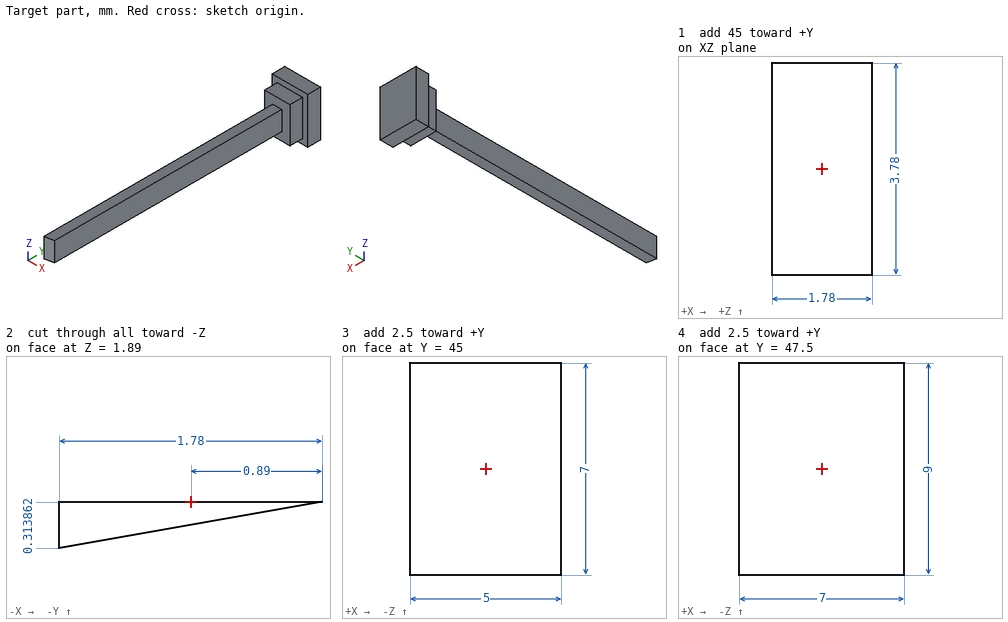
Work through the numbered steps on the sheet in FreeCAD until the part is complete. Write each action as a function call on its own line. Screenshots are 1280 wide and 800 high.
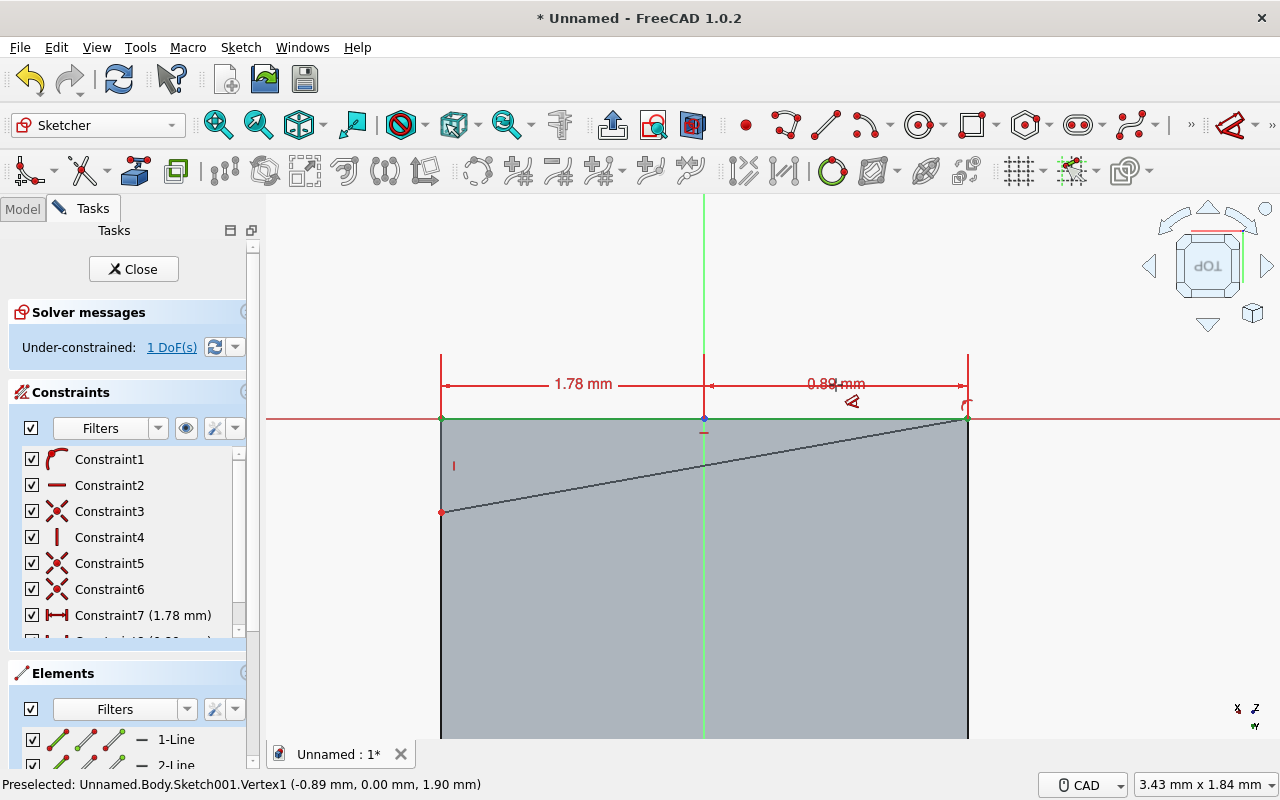
click(441, 447)
click(407, 466)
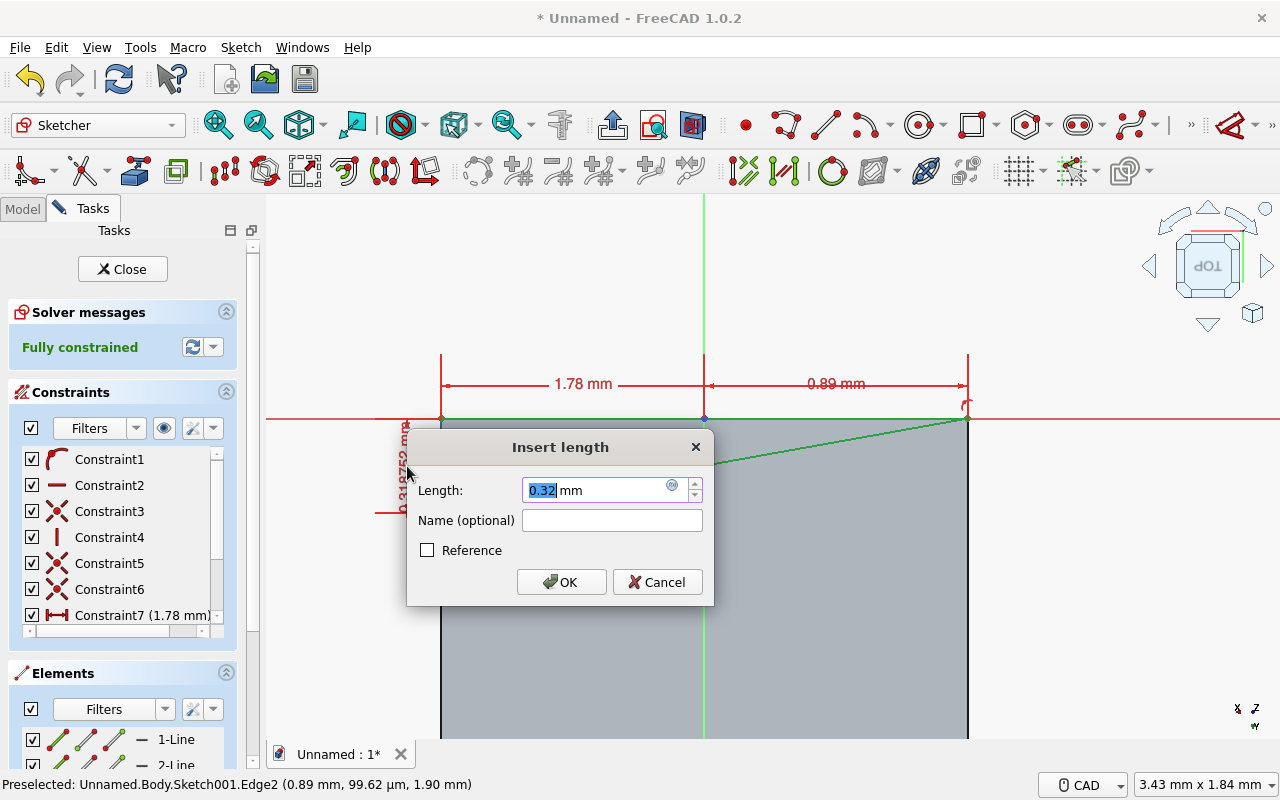
text(0.313862)
key(Return)
key(Escape)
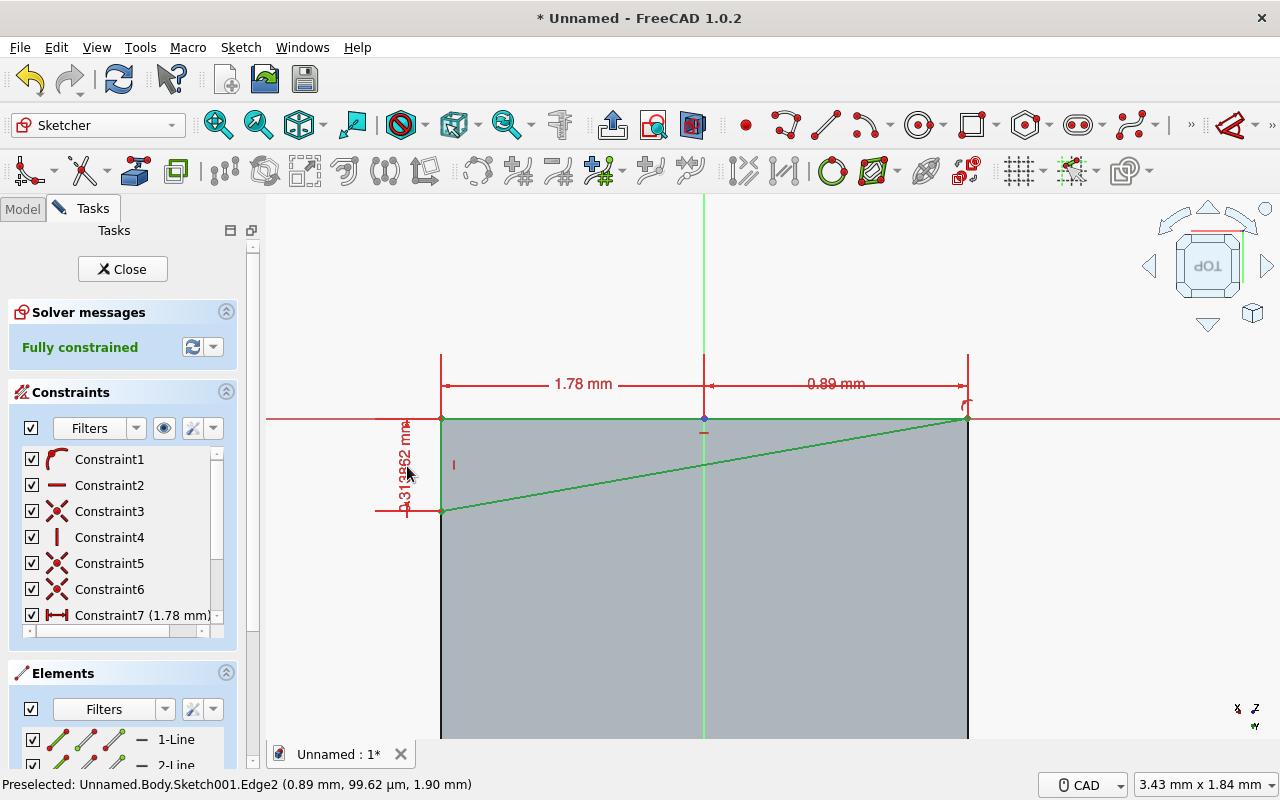
click(123, 269)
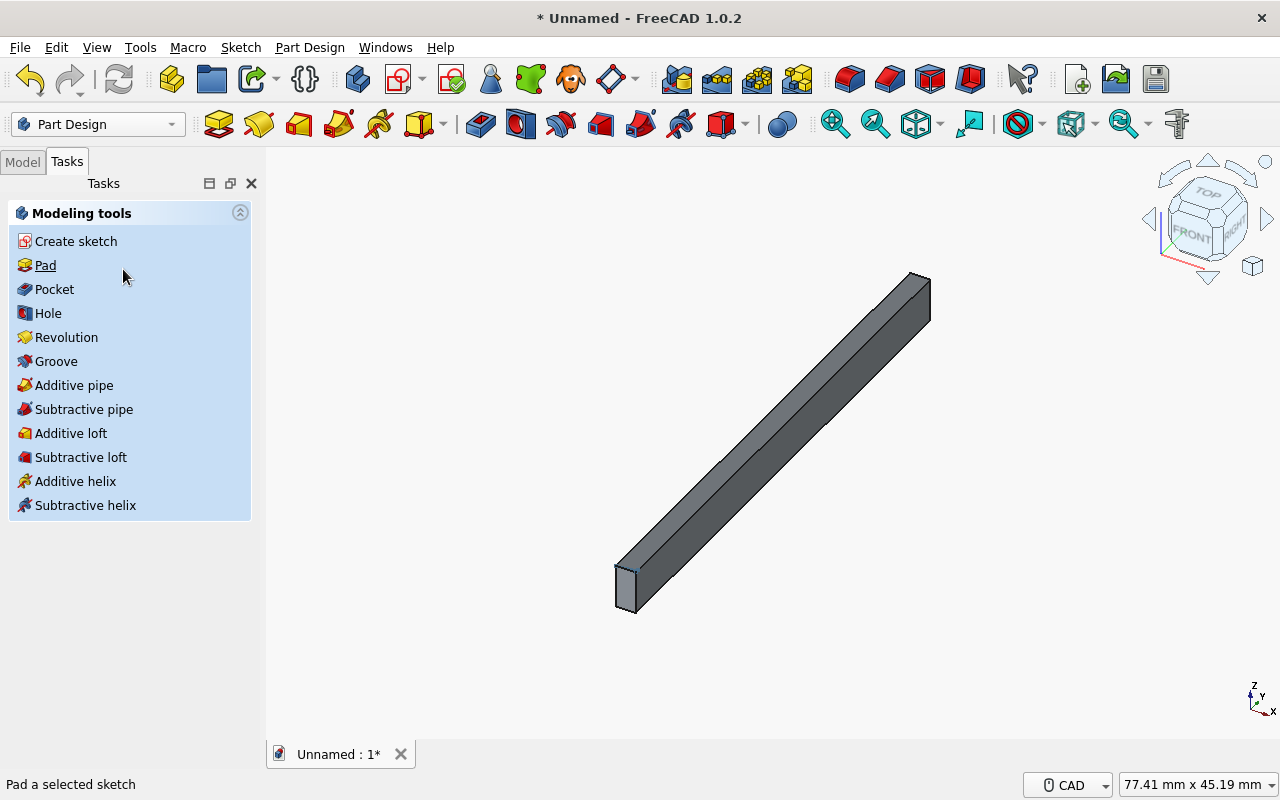
click(482, 124)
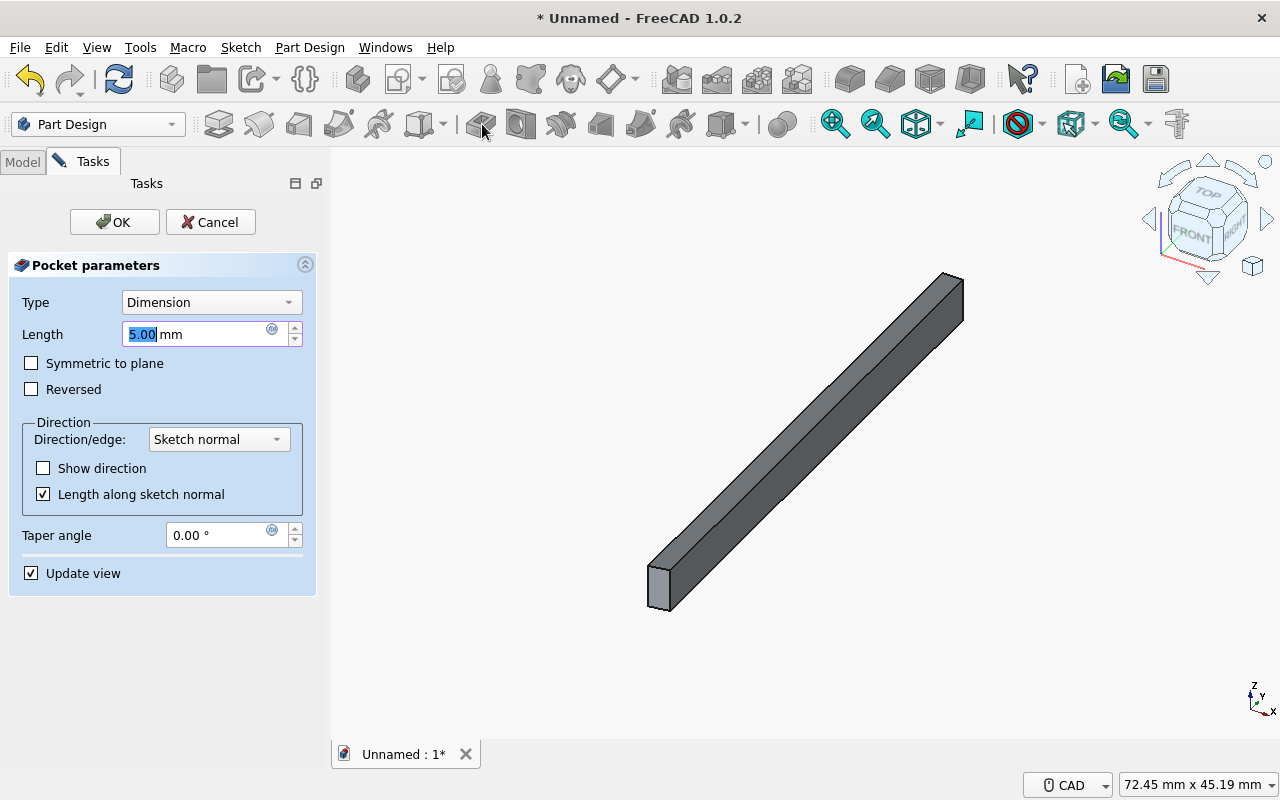
click(212, 302)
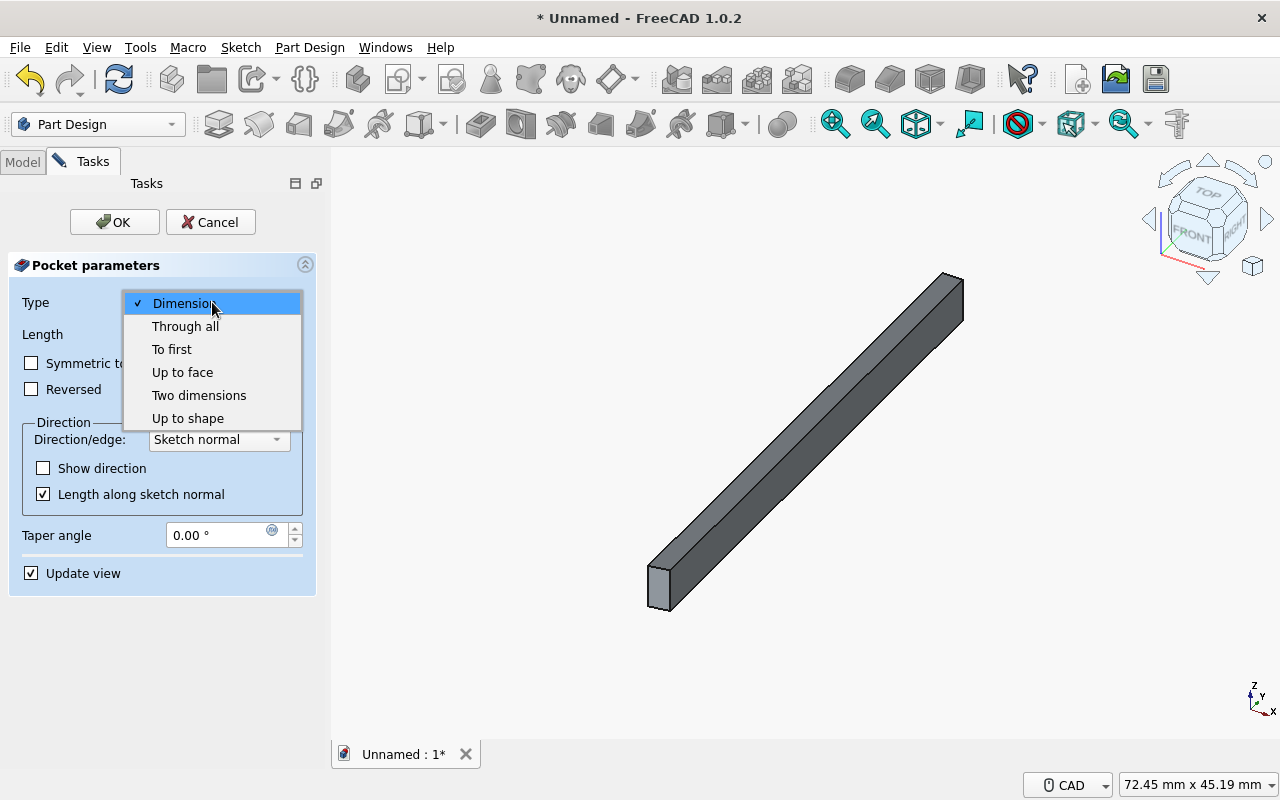
click(212, 326)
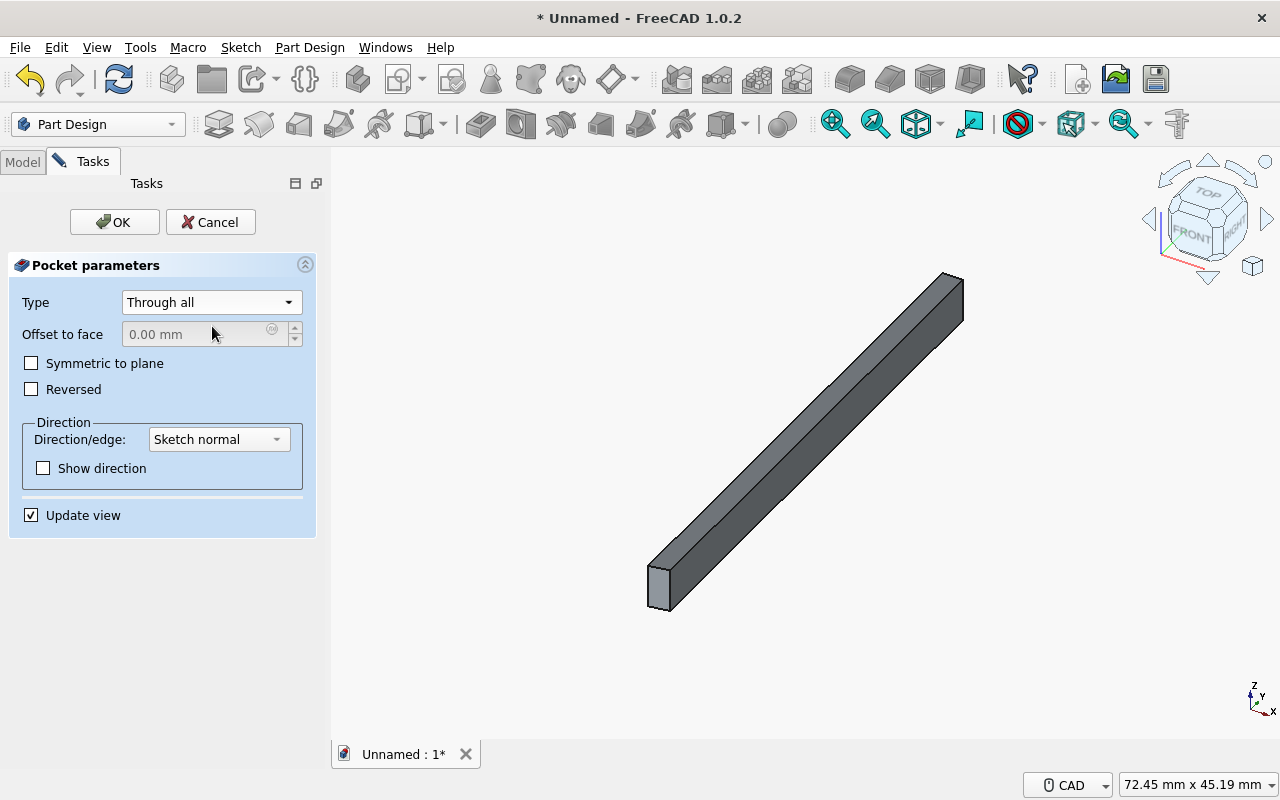
click(115, 222)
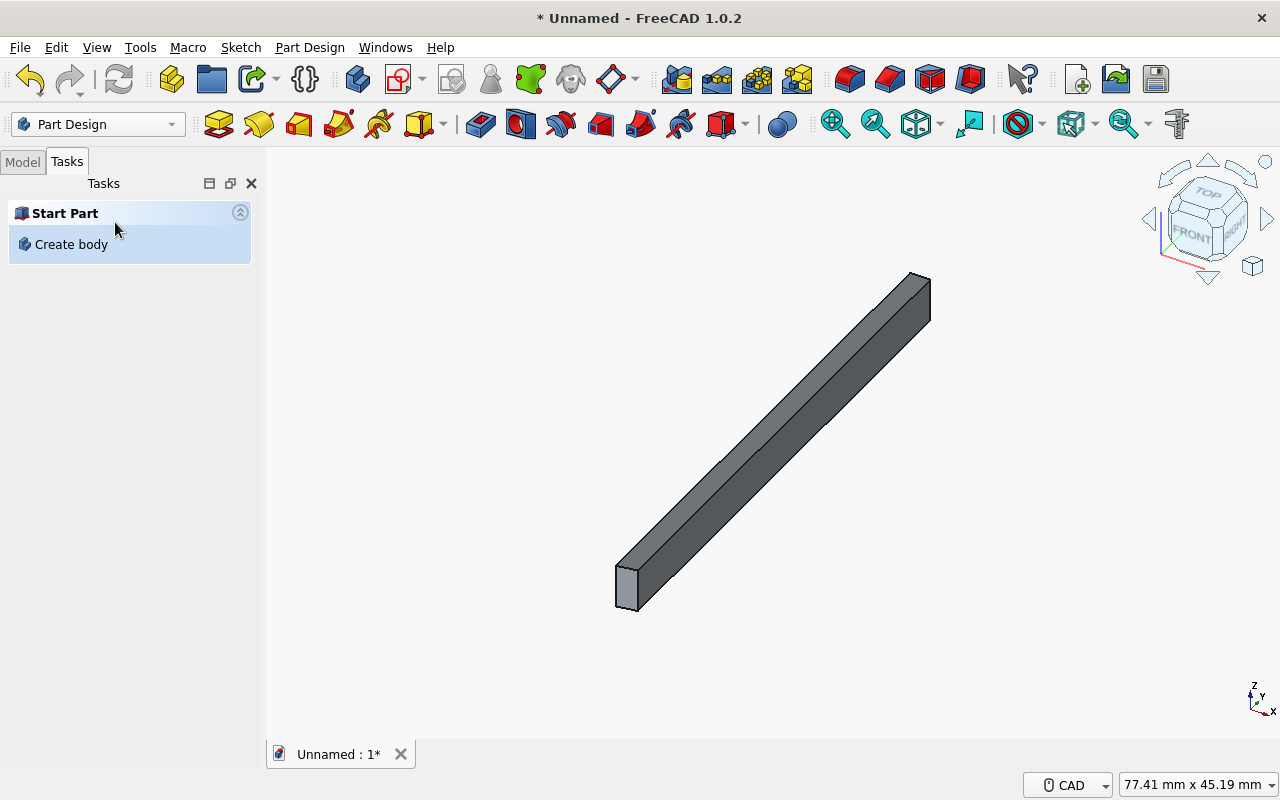
key(4)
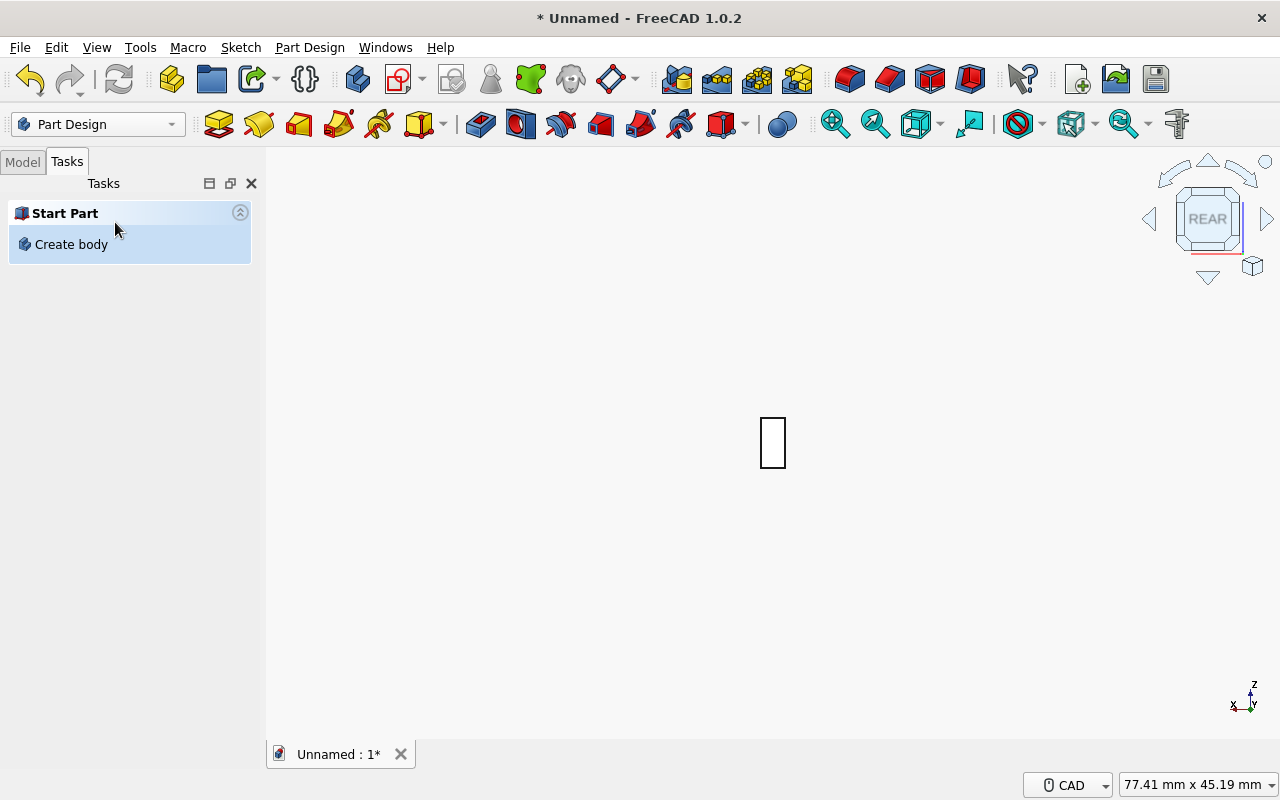
key(v)
key(f)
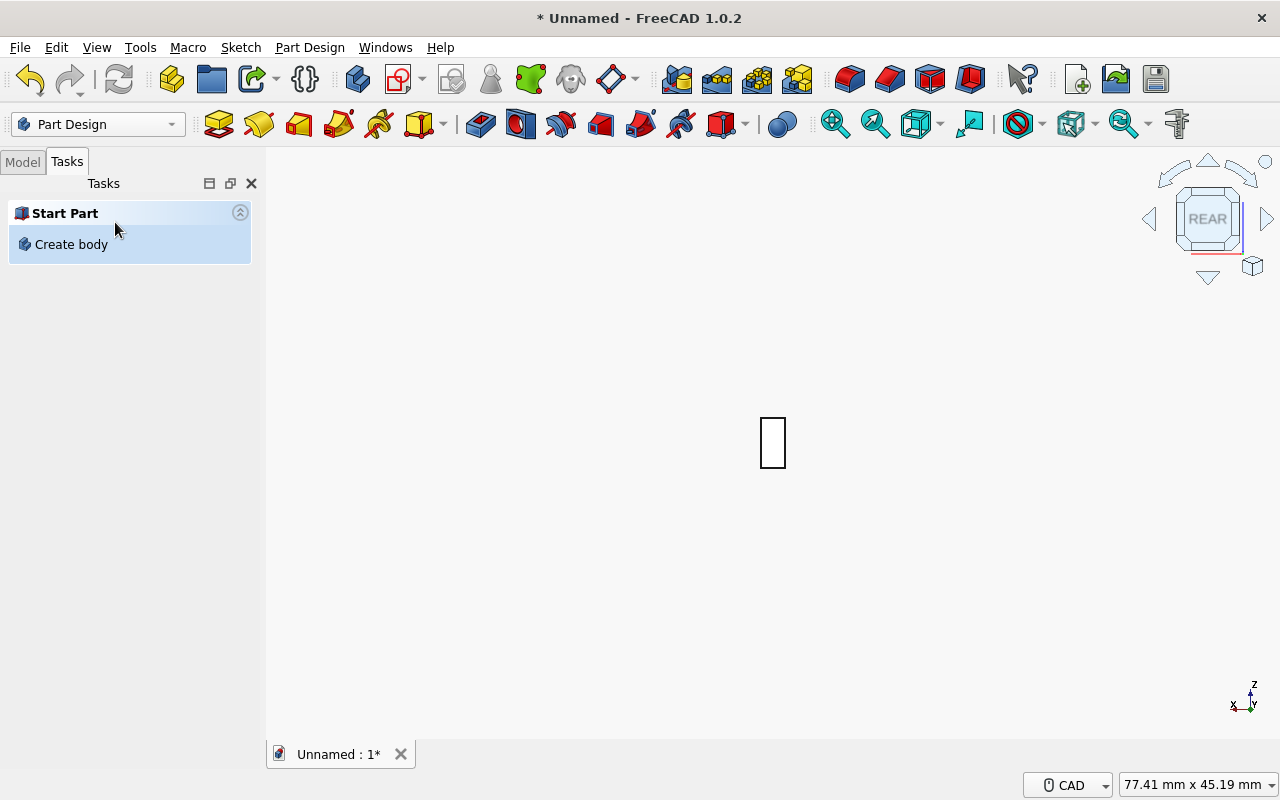
click(773, 435)